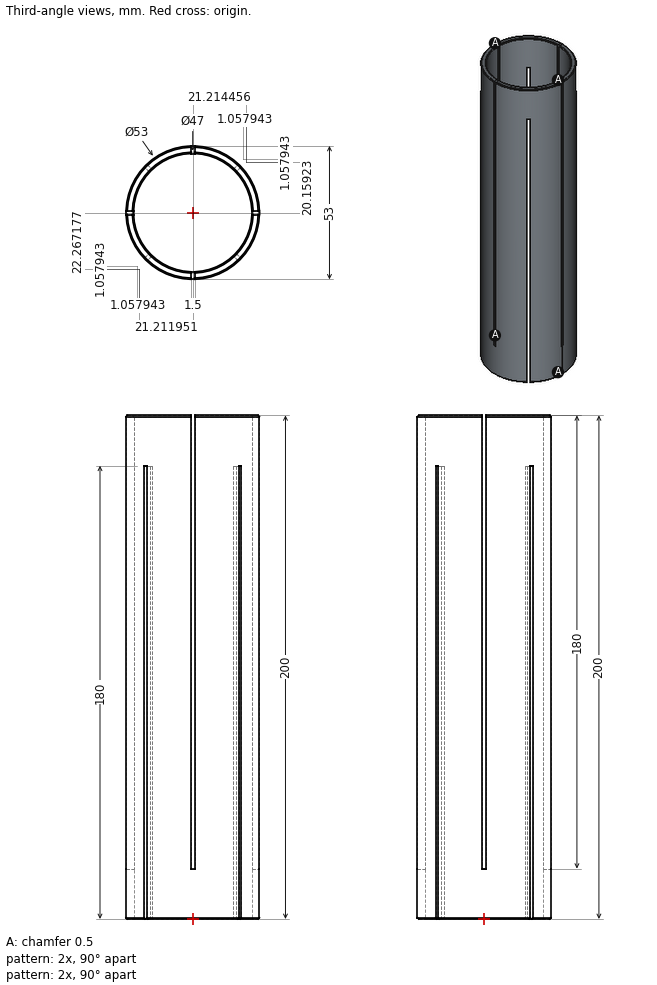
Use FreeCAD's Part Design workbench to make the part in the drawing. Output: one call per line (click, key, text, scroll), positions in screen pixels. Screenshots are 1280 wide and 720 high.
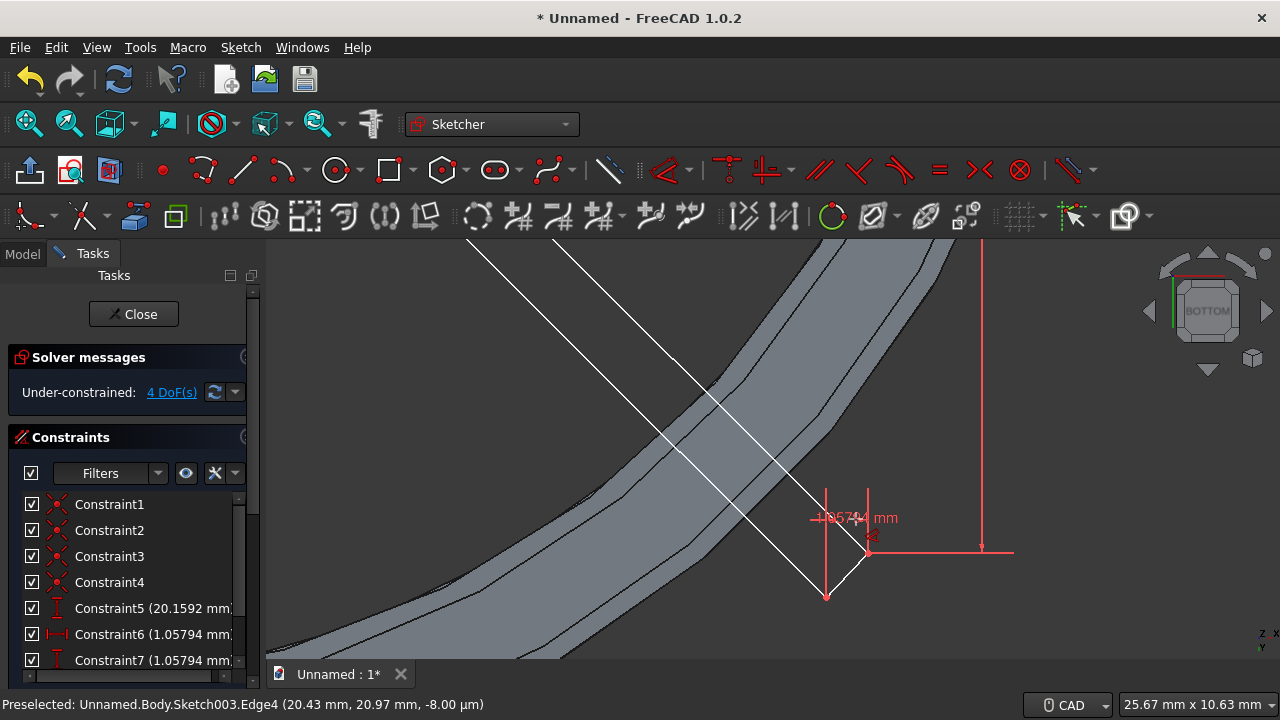
click(839, 585)
click(902, 576)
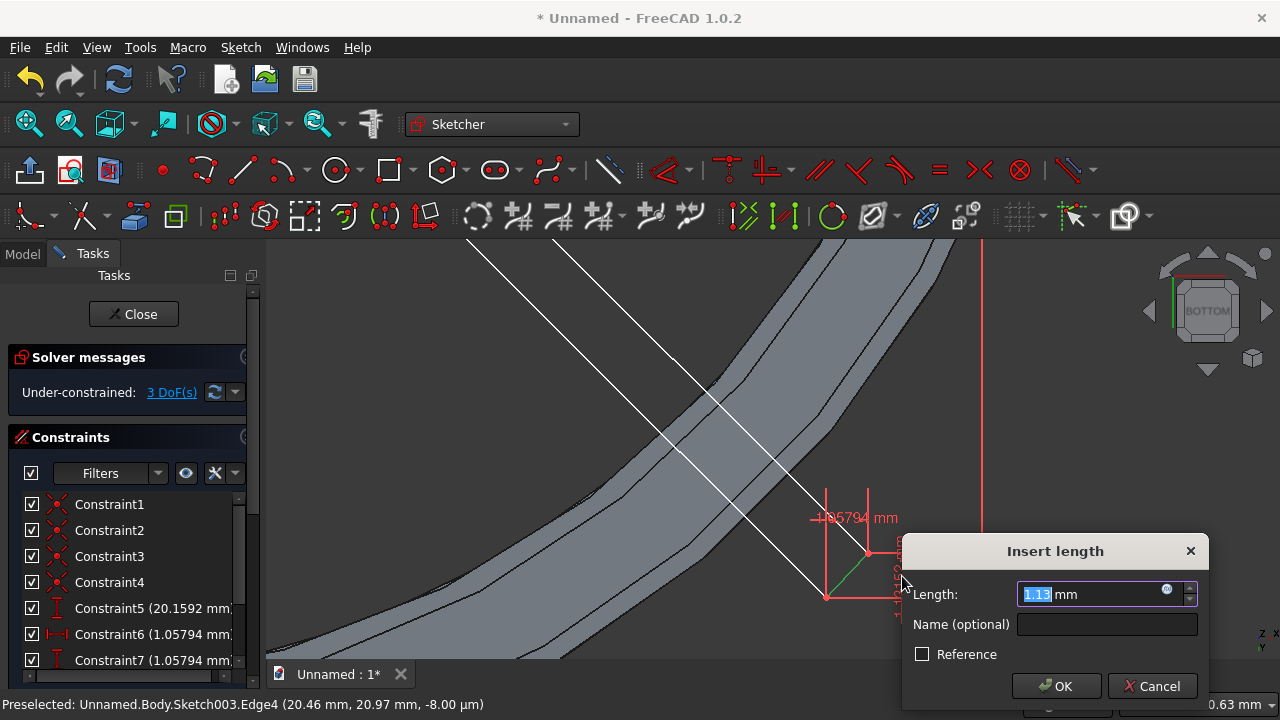
text(1.057943)
key(Return)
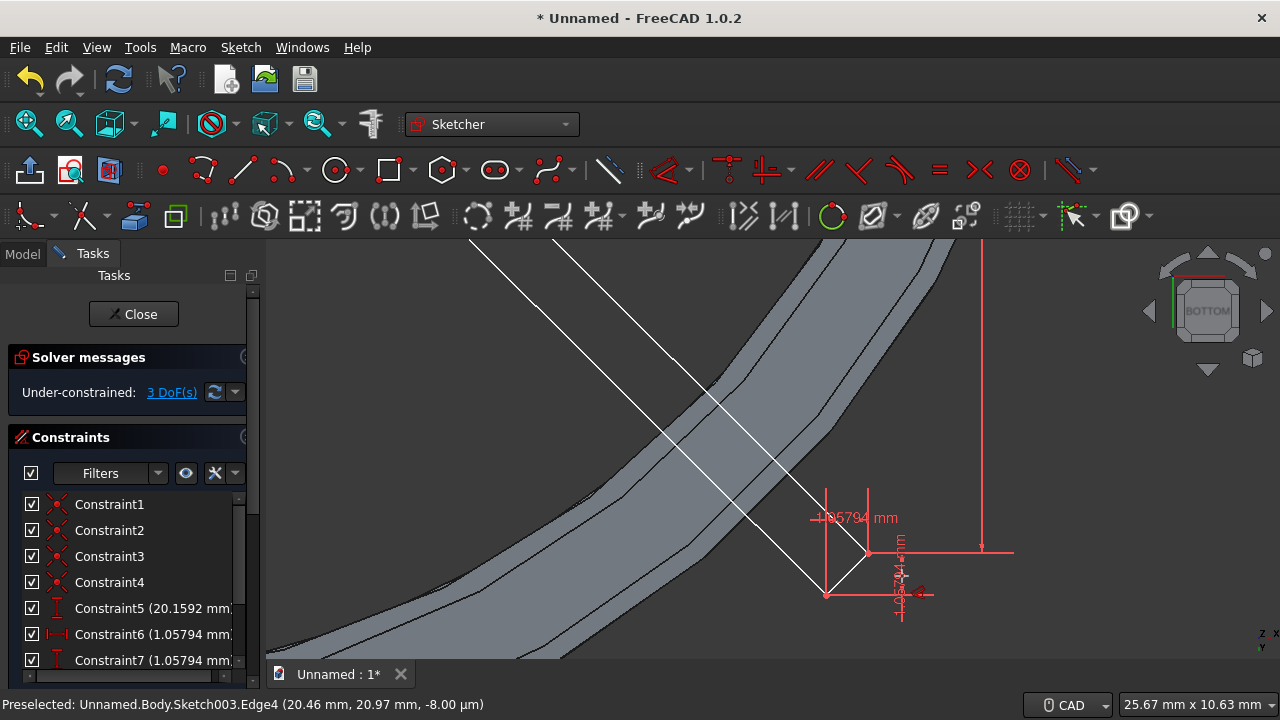
scroll(842, 590, down, 9)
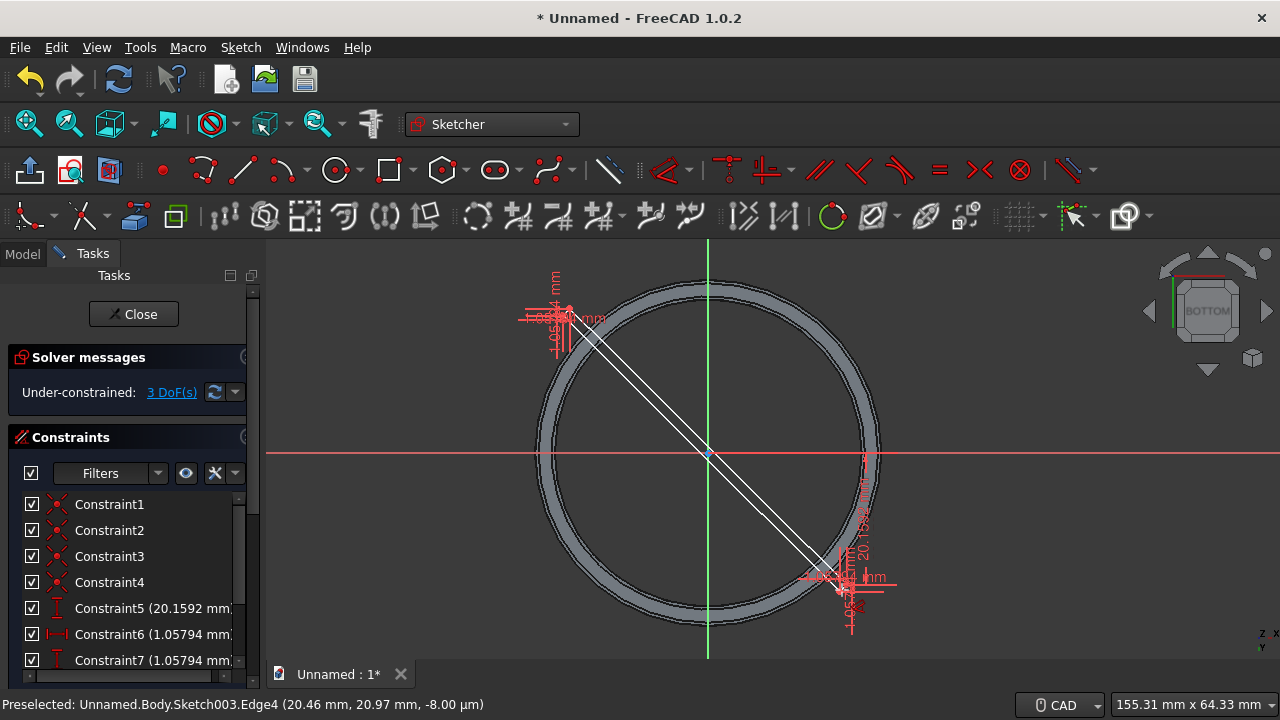
scroll(847, 585, up, 2)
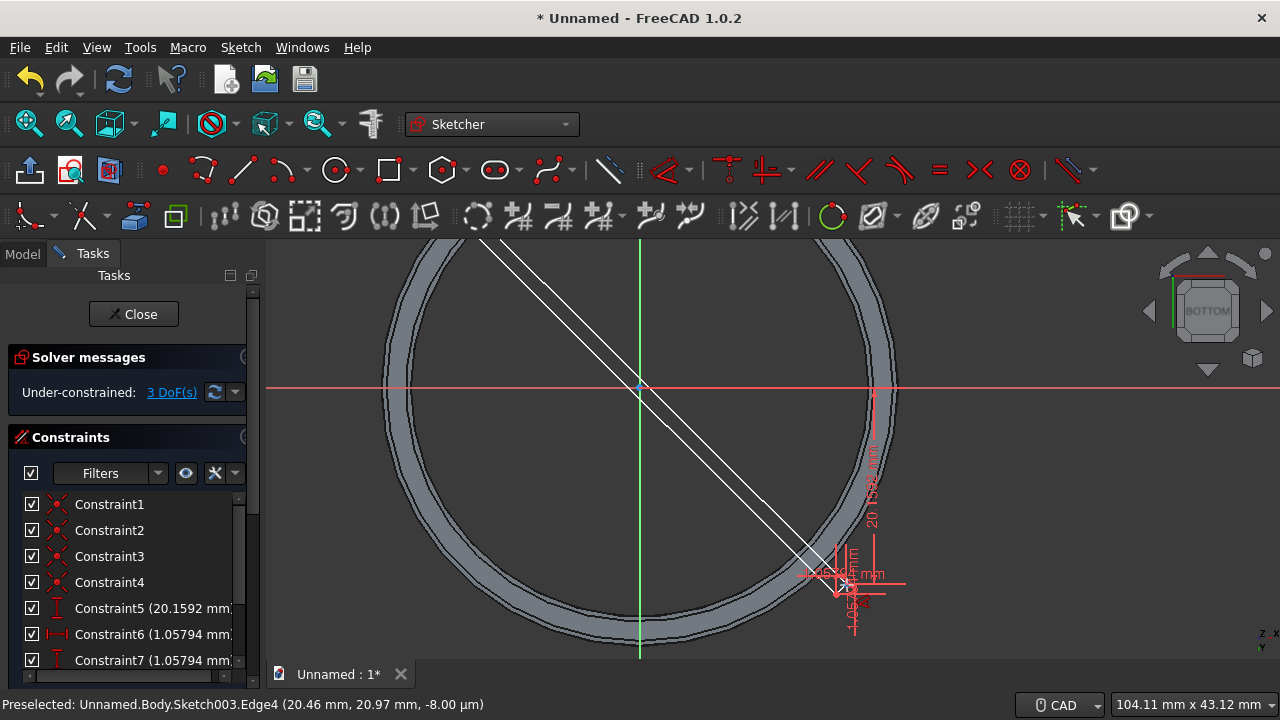
click(846, 584)
click(743, 618)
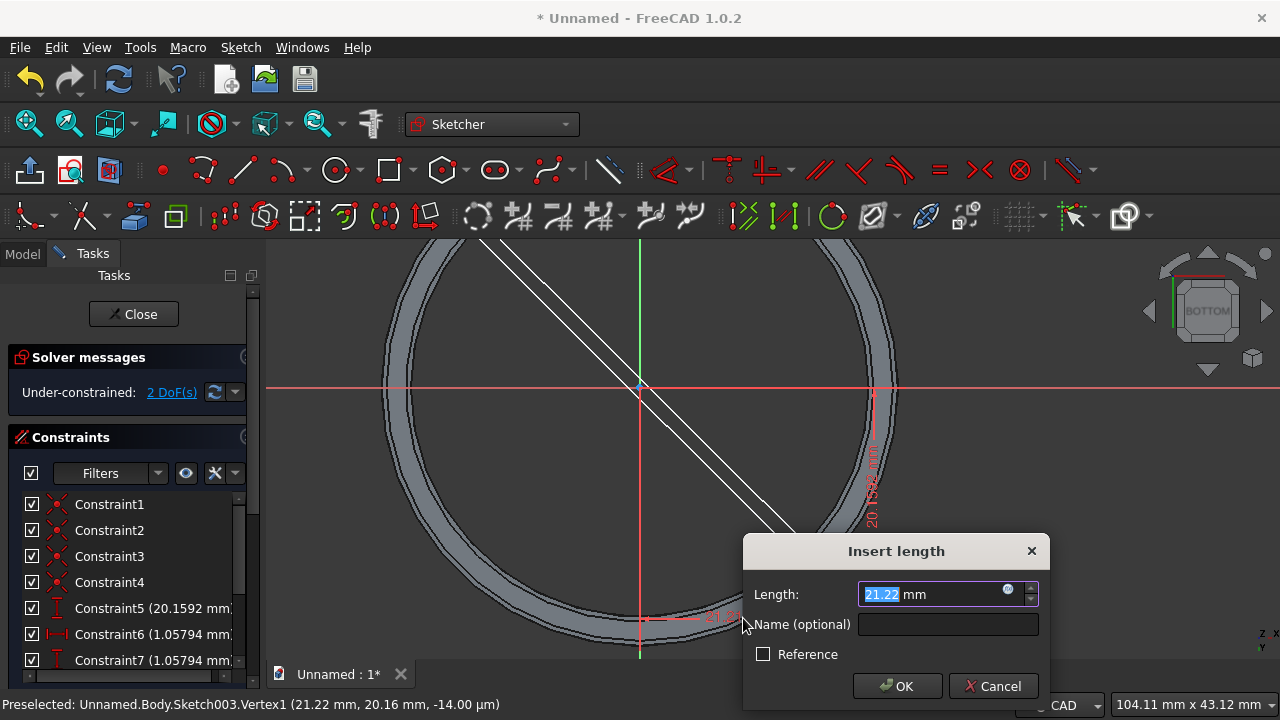
text(21.214456)
key(Return)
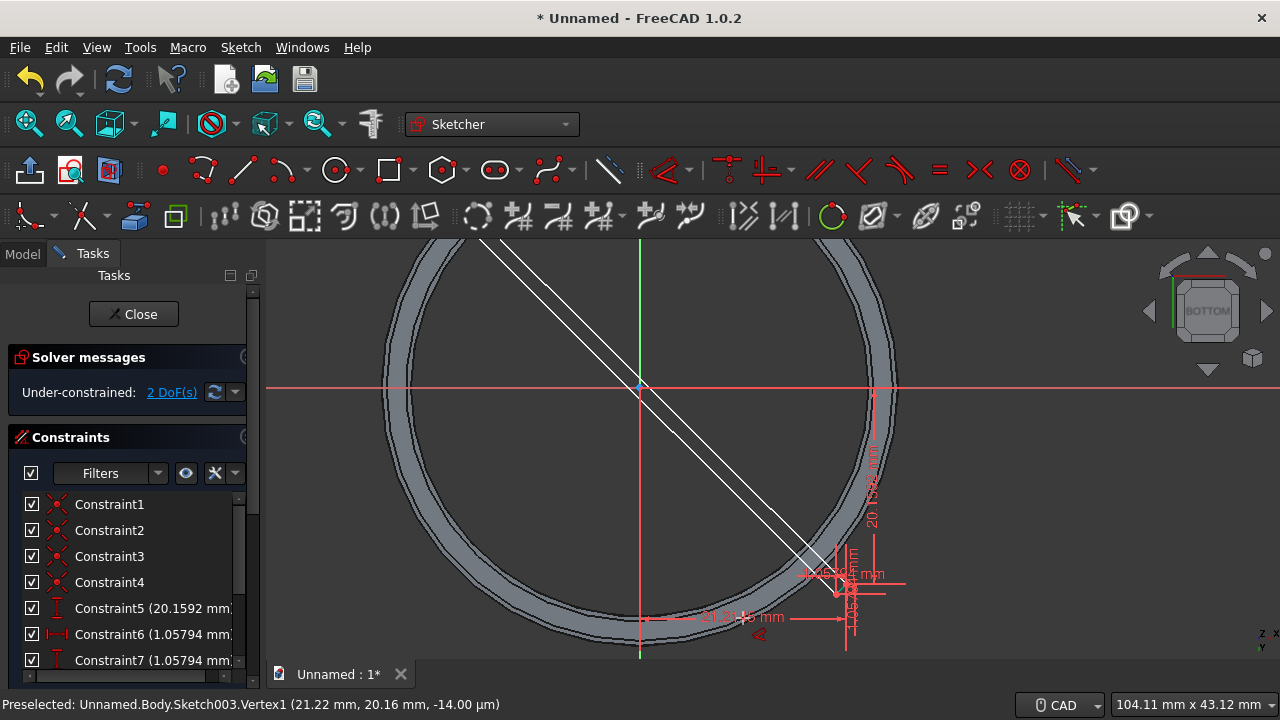
scroll(847, 584, down, 2)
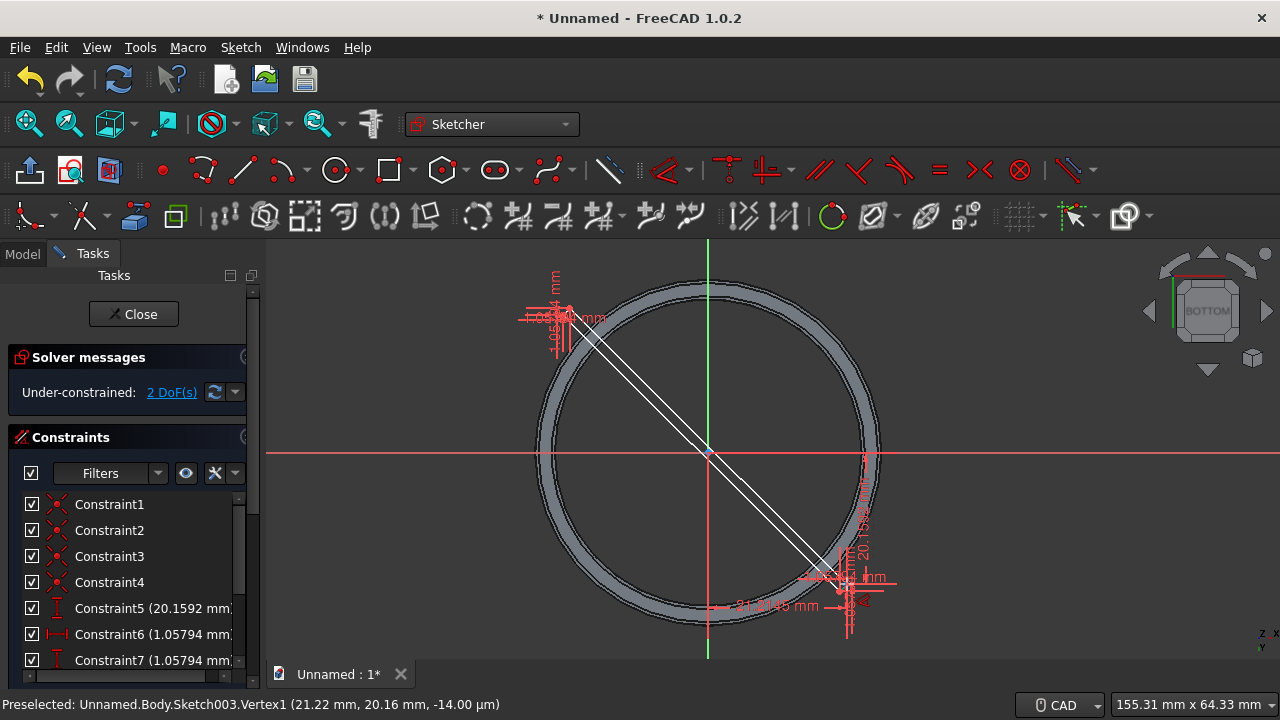
scroll(570, 308, up, 2)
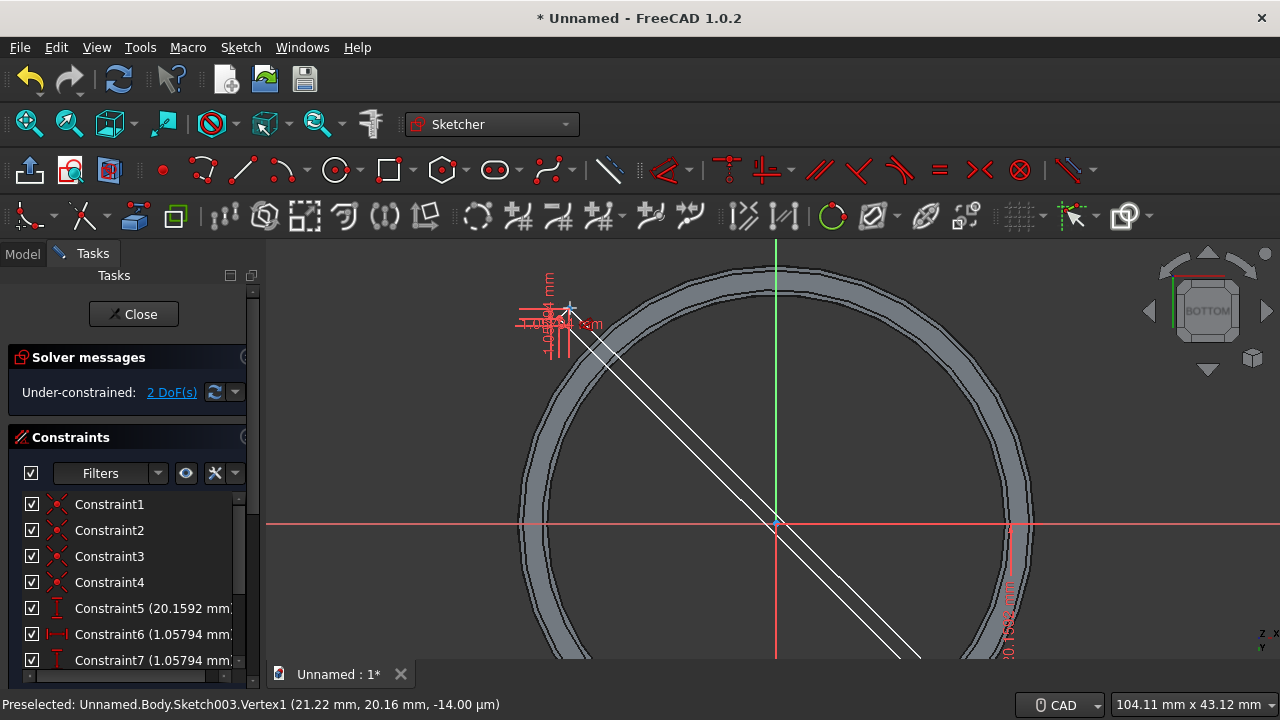
click(569, 309)
click(673, 275)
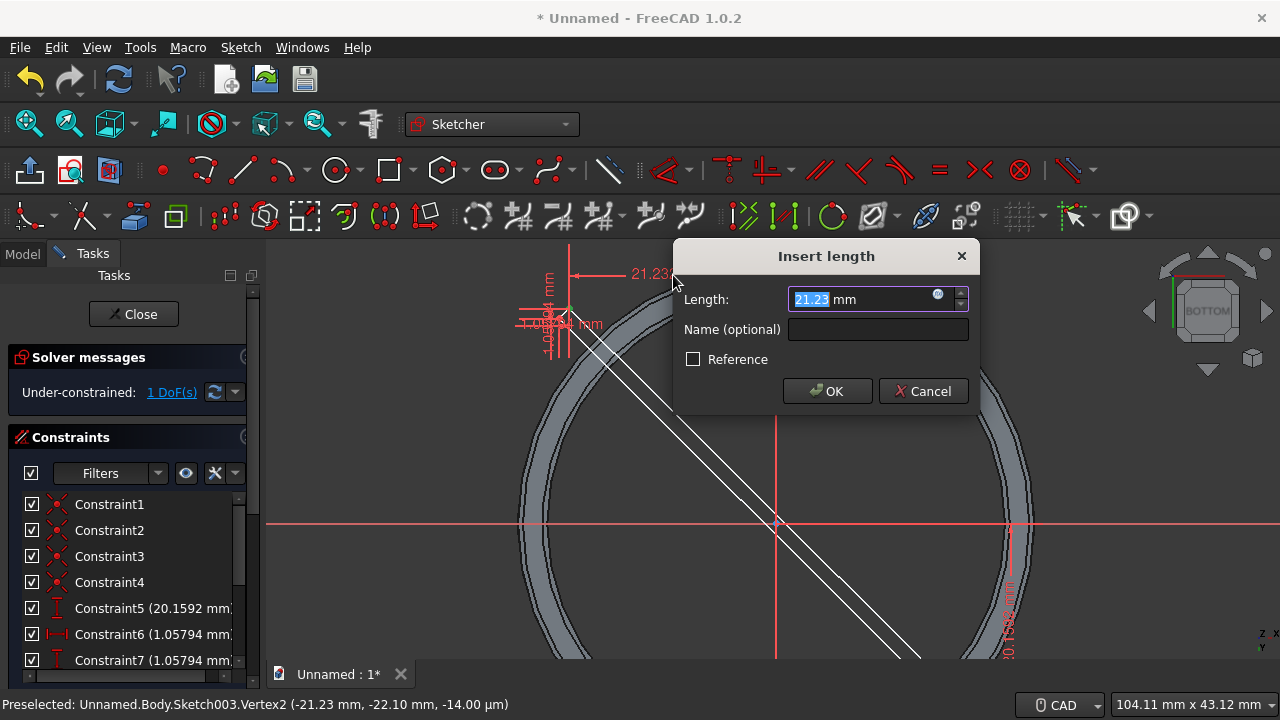
text(21.211951)
key(Return)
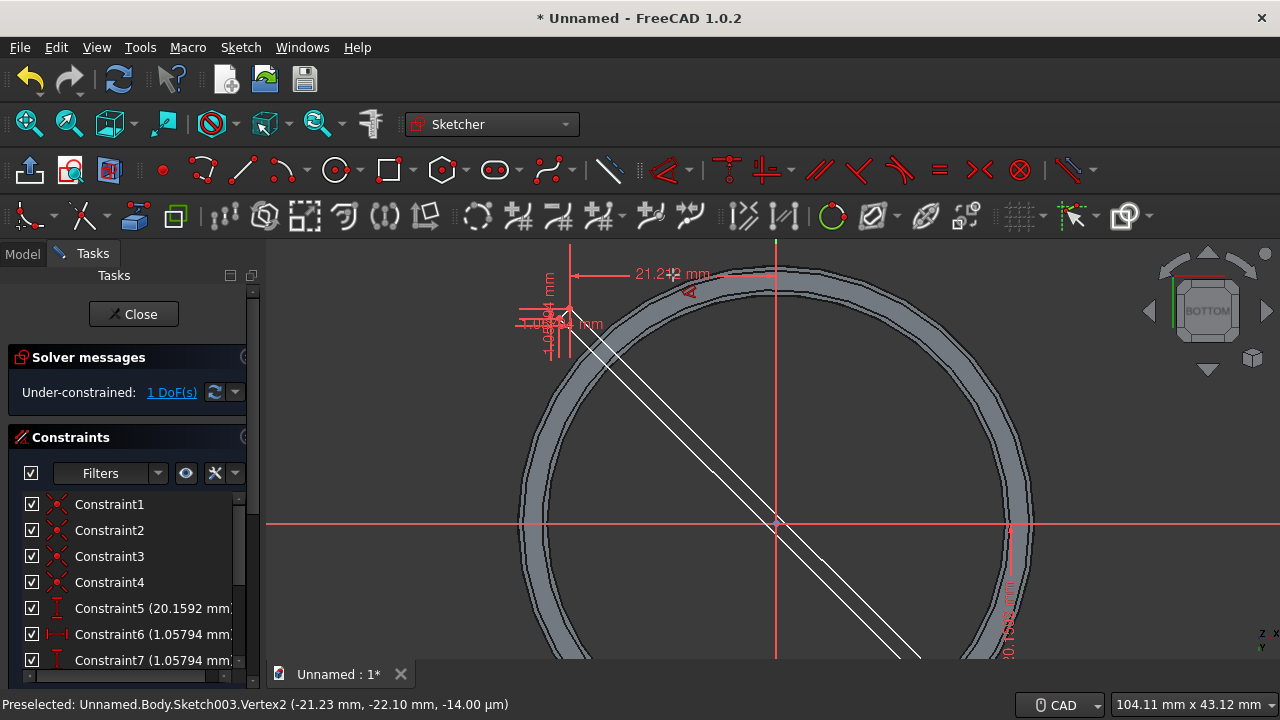
click(570, 309)
click(536, 416)